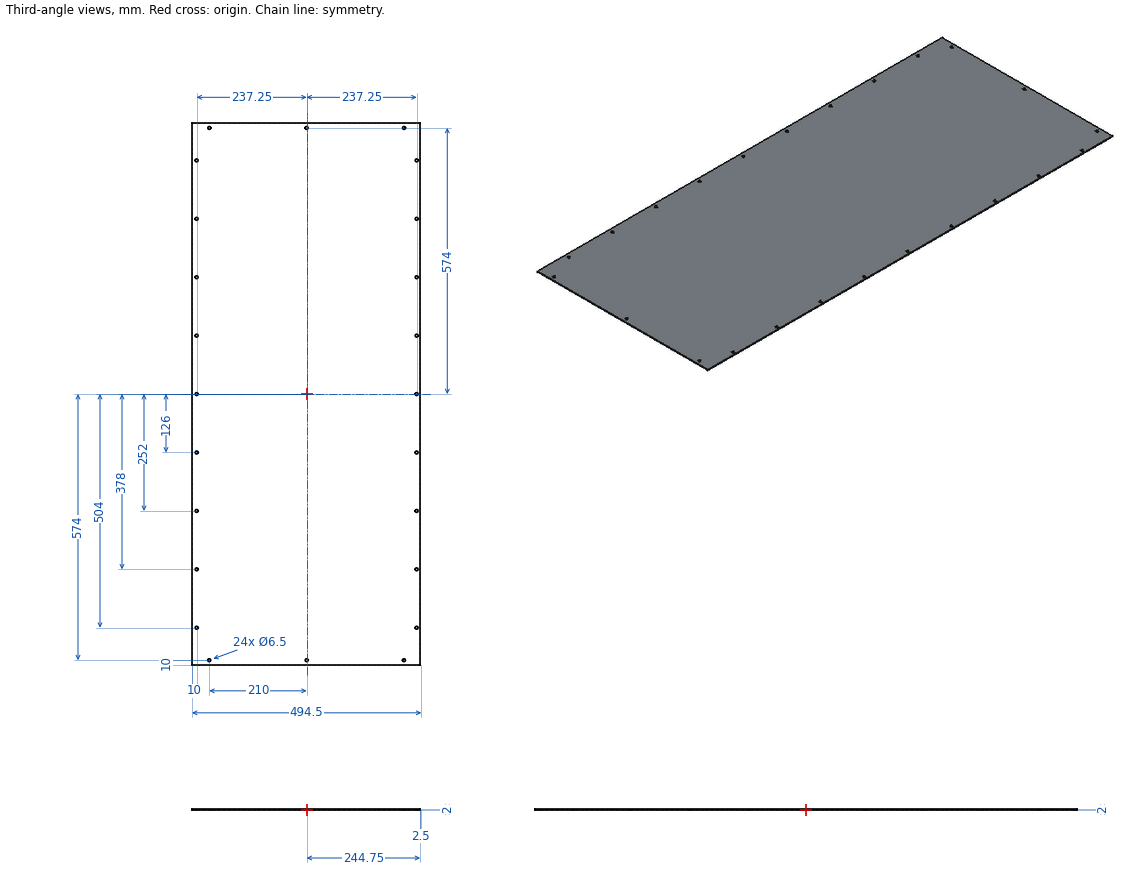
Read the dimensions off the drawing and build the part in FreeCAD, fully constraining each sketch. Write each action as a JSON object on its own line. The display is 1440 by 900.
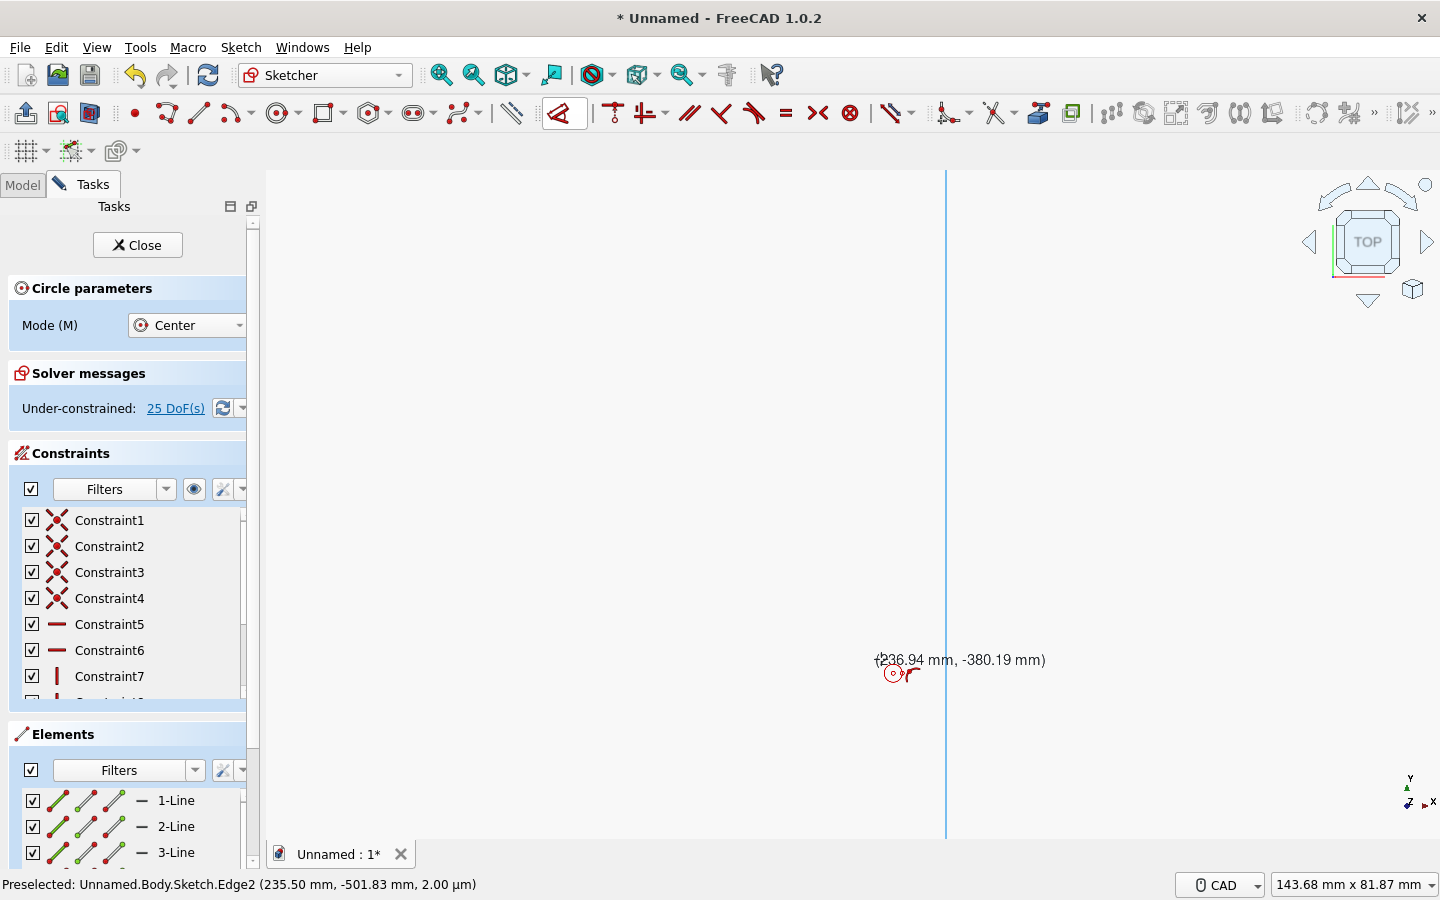
{"action": "scroll", "coordinate": [881, 659], "scroll_direction": "down", "scroll_amount": 15}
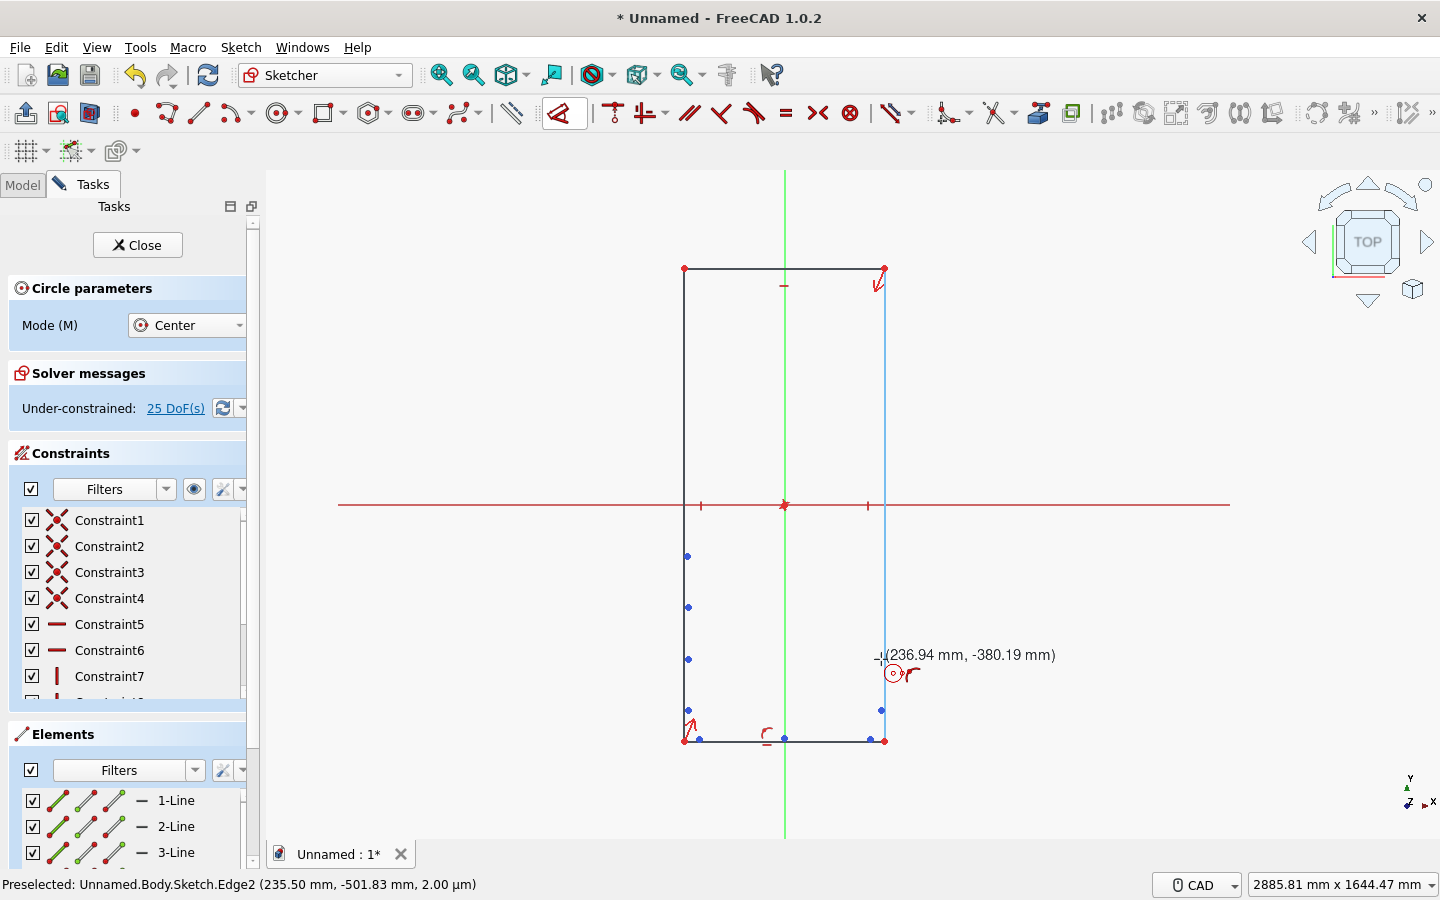
{"action": "scroll", "coordinate": [881, 659], "scroll_direction": "up", "scroll_amount": 7}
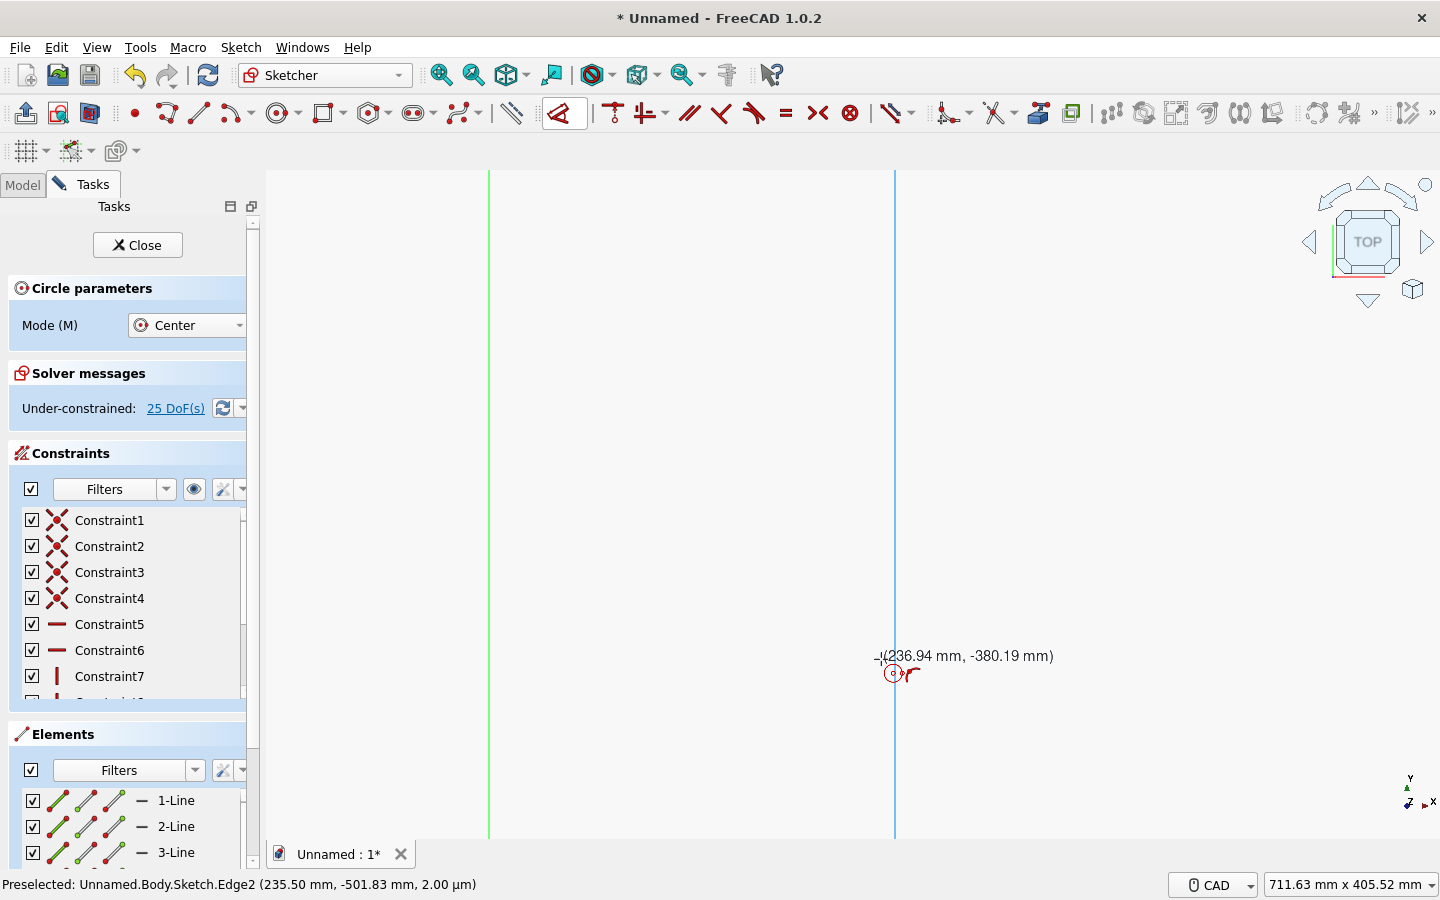
{"action": "left_click", "coordinate": [880, 657]}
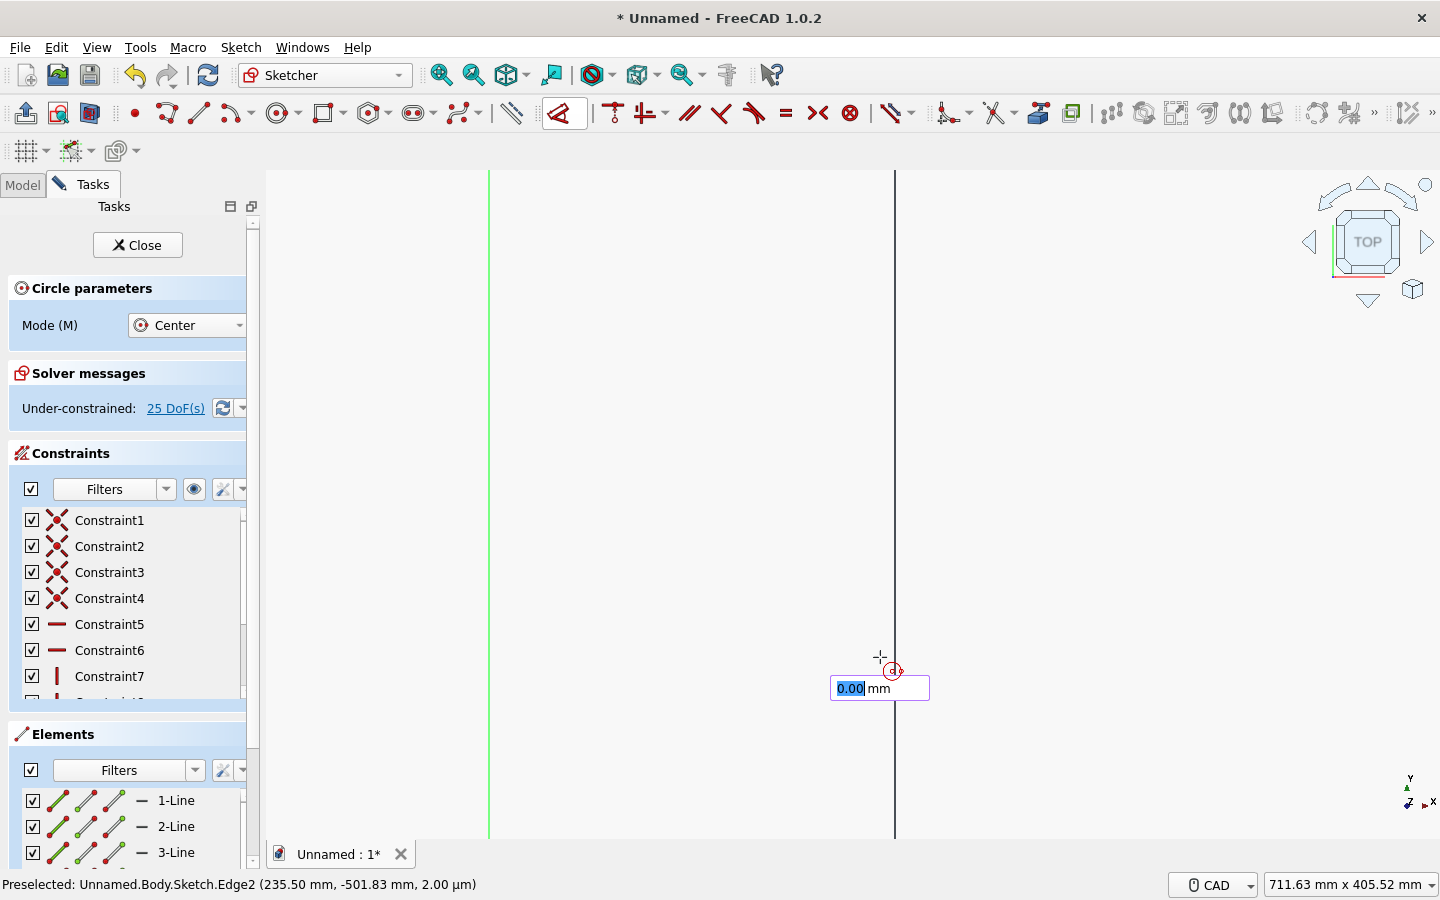
{"action": "scroll", "coordinate": [876, 653], "scroll_direction": "up", "scroll_amount": 6}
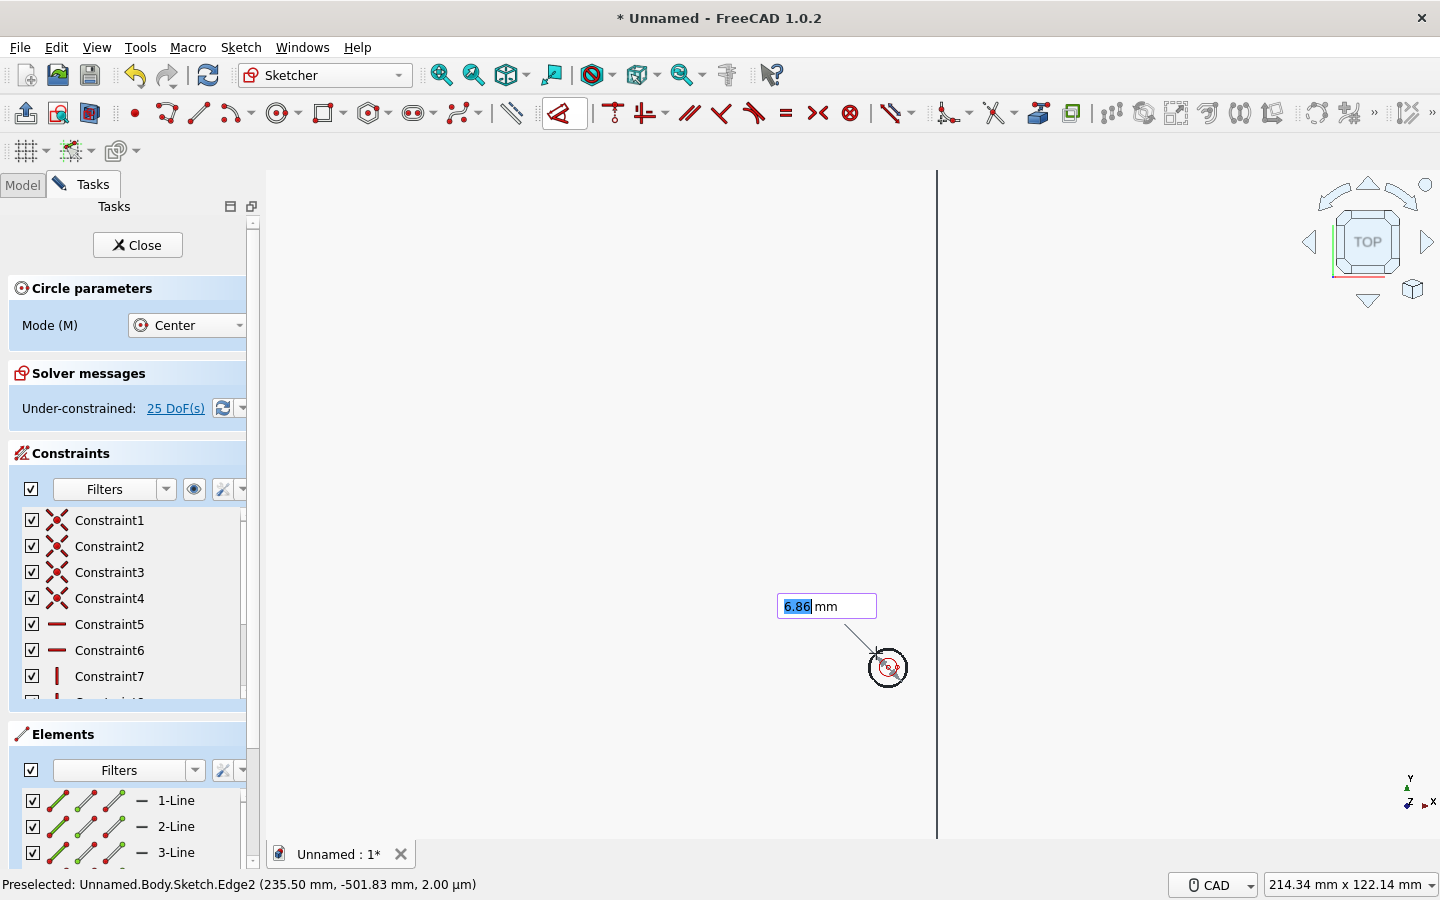
{"action": "left_click", "coordinate": [875, 653]}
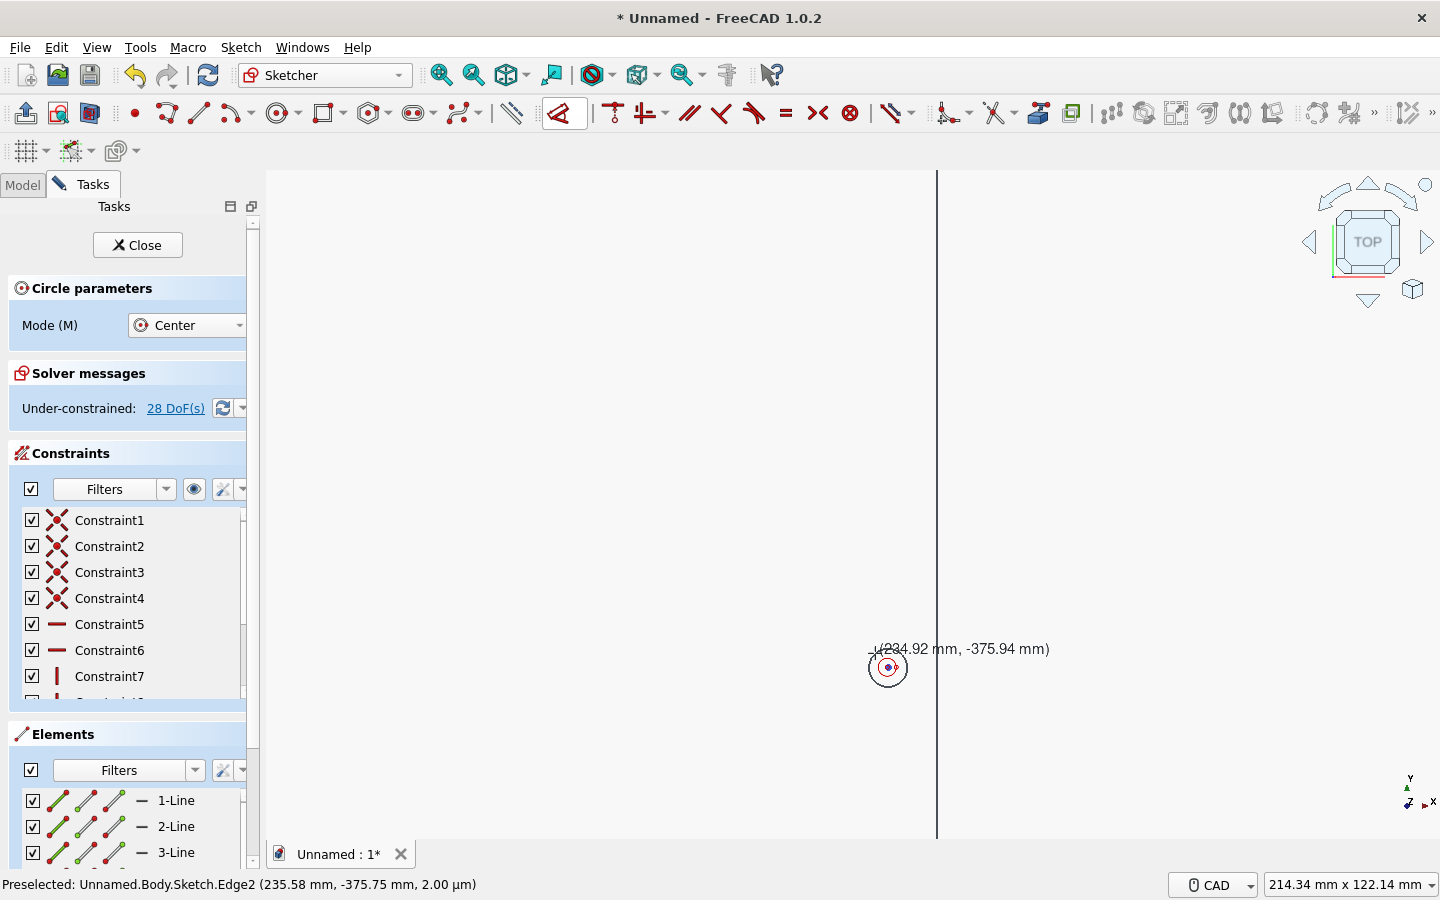
{"action": "scroll", "coordinate": [880, 658], "scroll_direction": "down", "scroll_amount": 13}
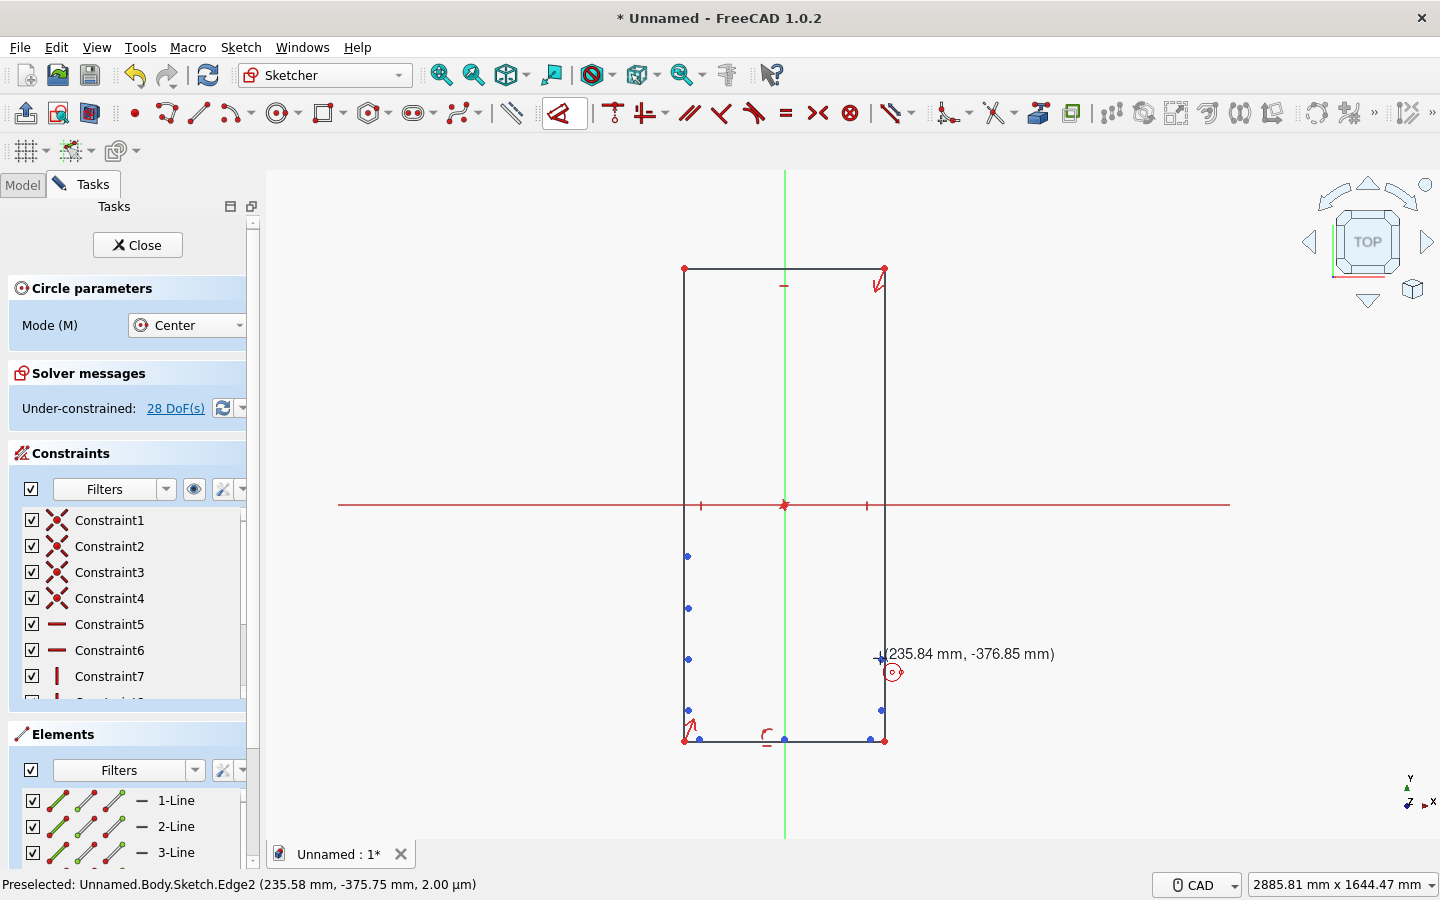
{"action": "scroll", "coordinate": [881, 608], "scroll_direction": "up", "scroll_amount": 15}